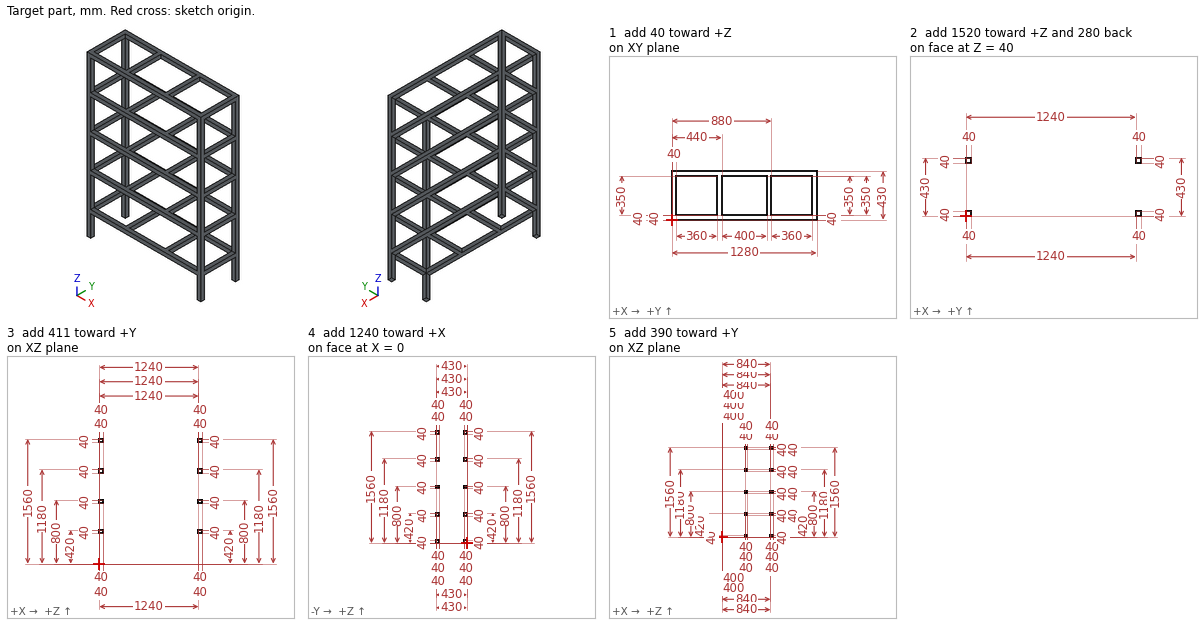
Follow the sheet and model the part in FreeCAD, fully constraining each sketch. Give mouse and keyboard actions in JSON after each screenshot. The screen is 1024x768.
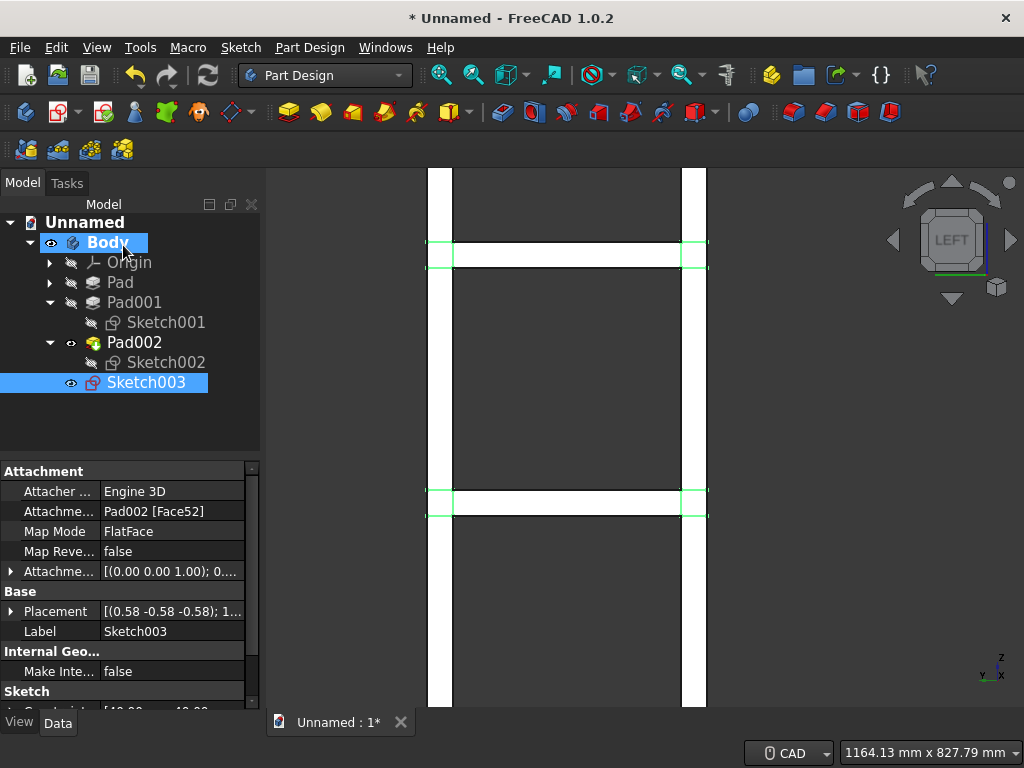
{"action": "left_click", "coordinate": [290, 112]}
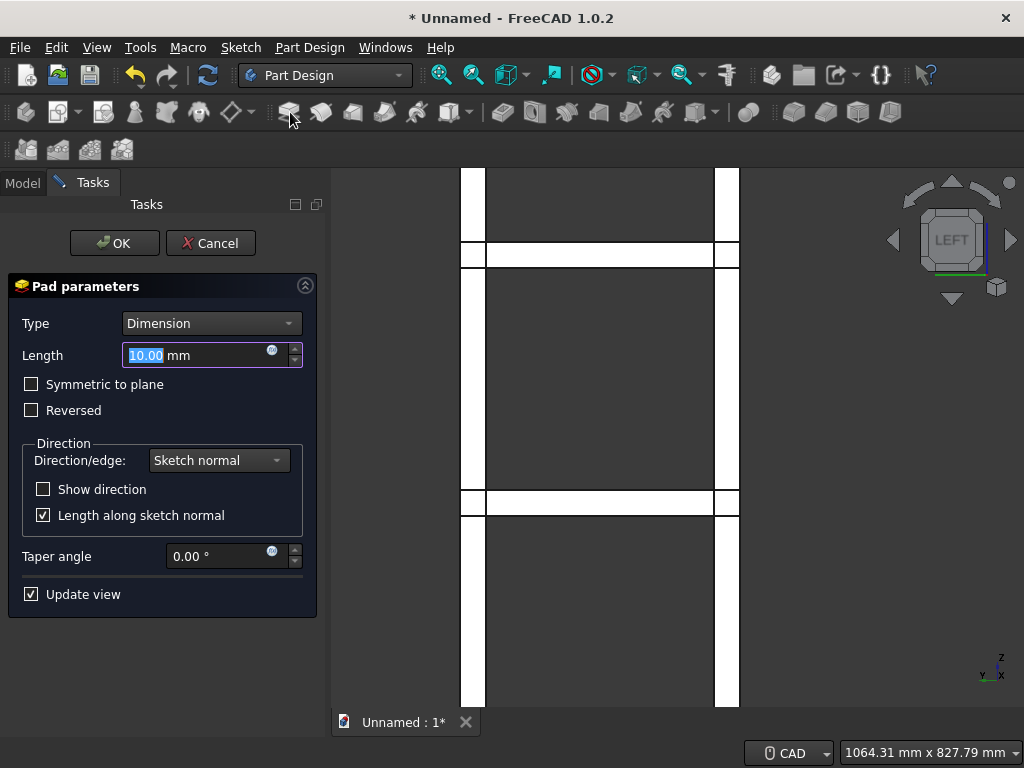
{"action": "type", "text": "1240"}
{"action": "key", "text": "Tab"}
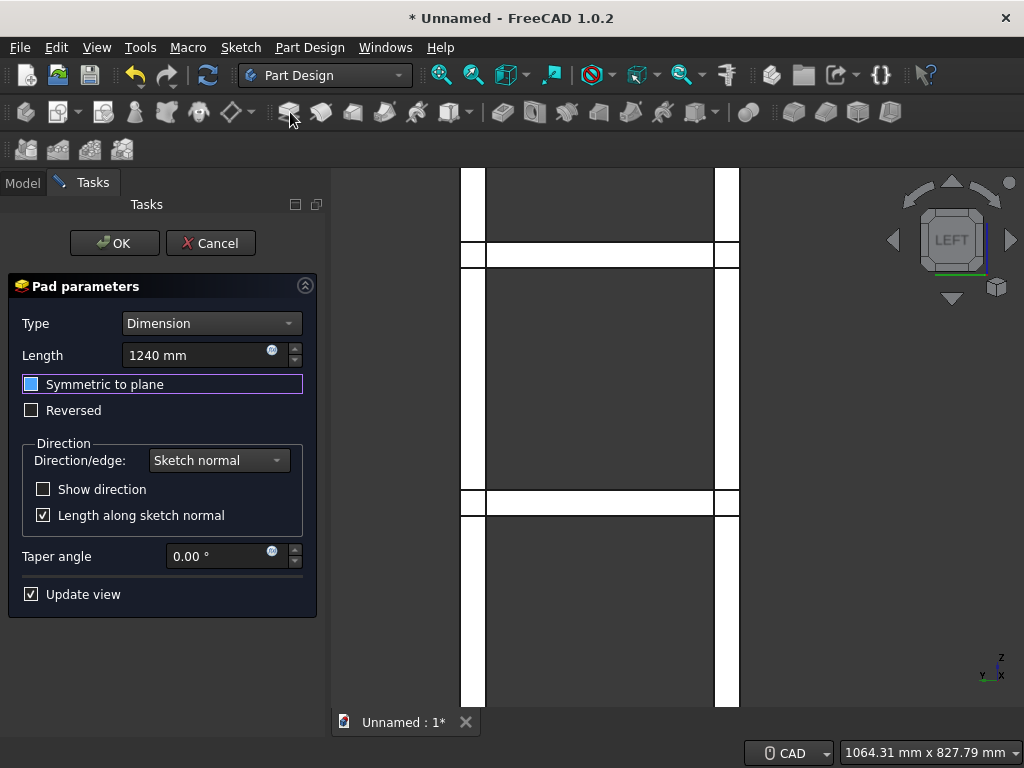
{"action": "left_click", "coordinate": [30, 410]}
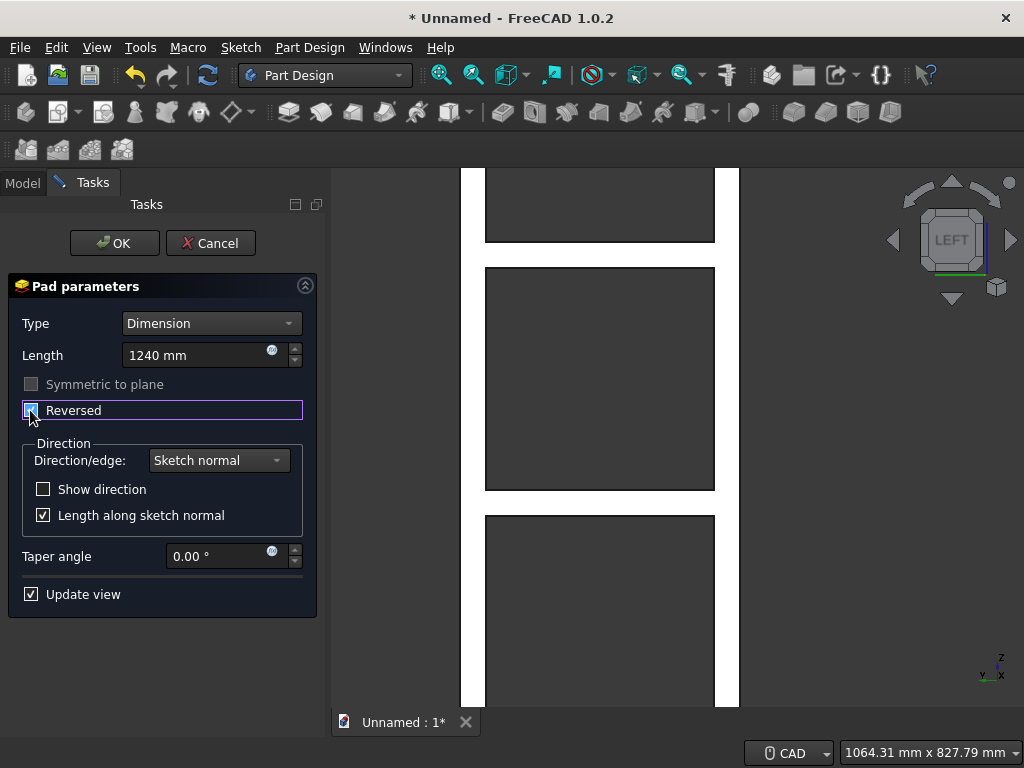
{"action": "left_click", "coordinate": [115, 243]}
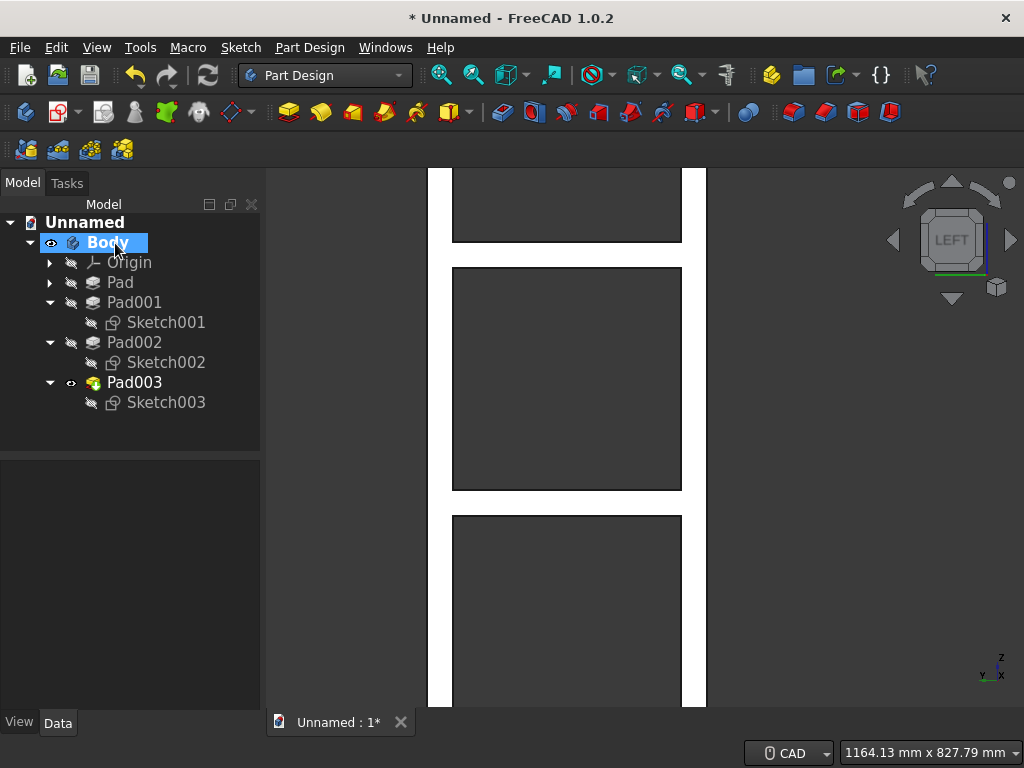
{"action": "left_click", "coordinate": [442, 76]}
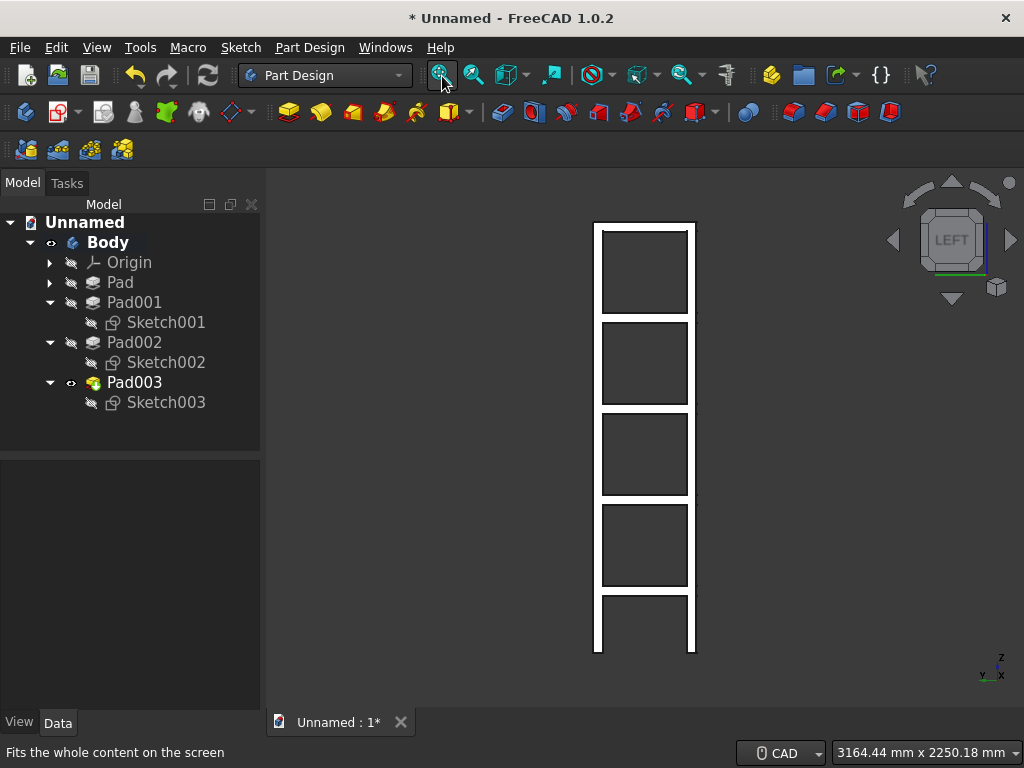
{"action": "left_click", "coordinate": [58, 112]}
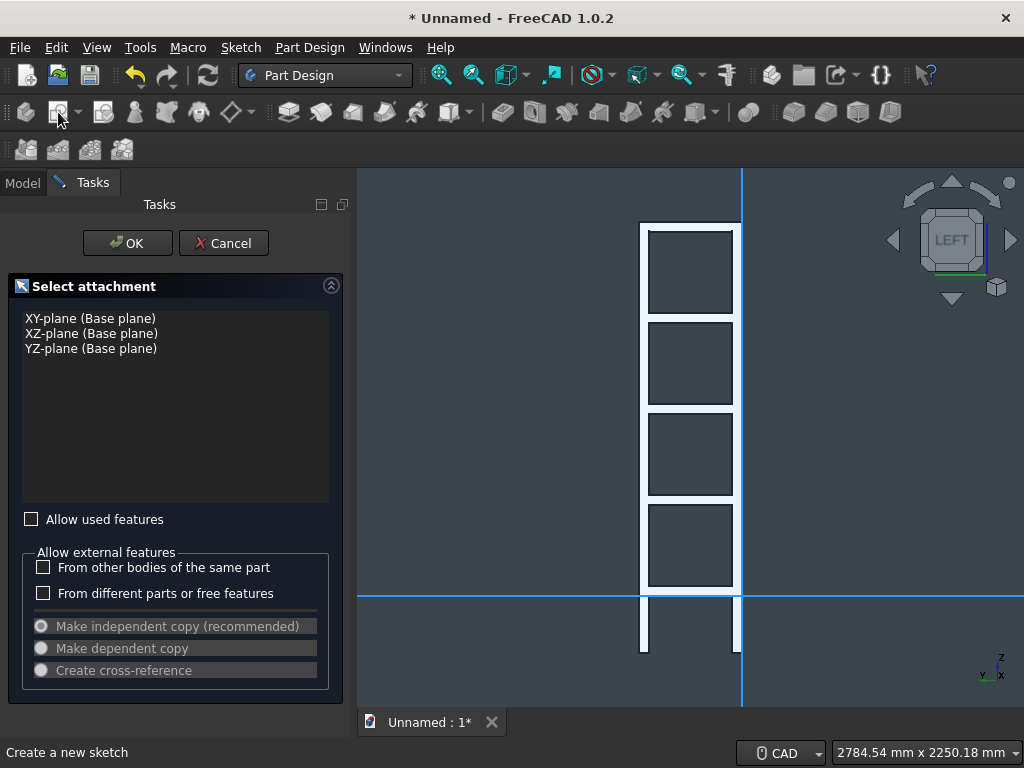
{"action": "left_click", "coordinate": [82, 334]}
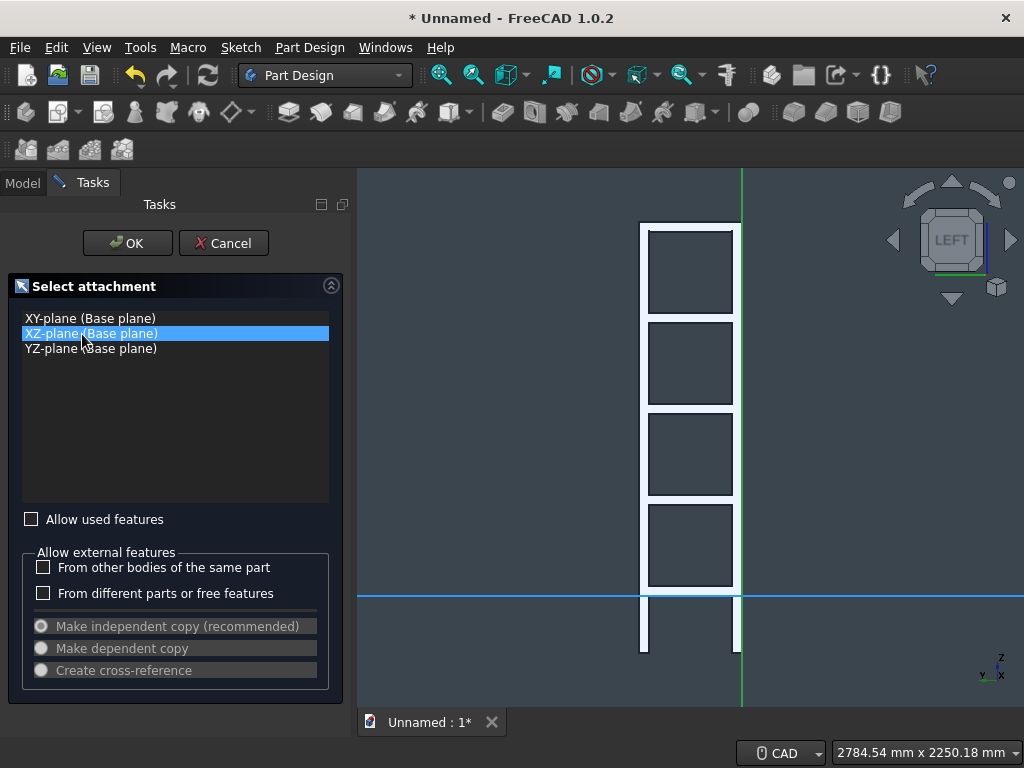
{"action": "left_click", "coordinate": [128, 243]}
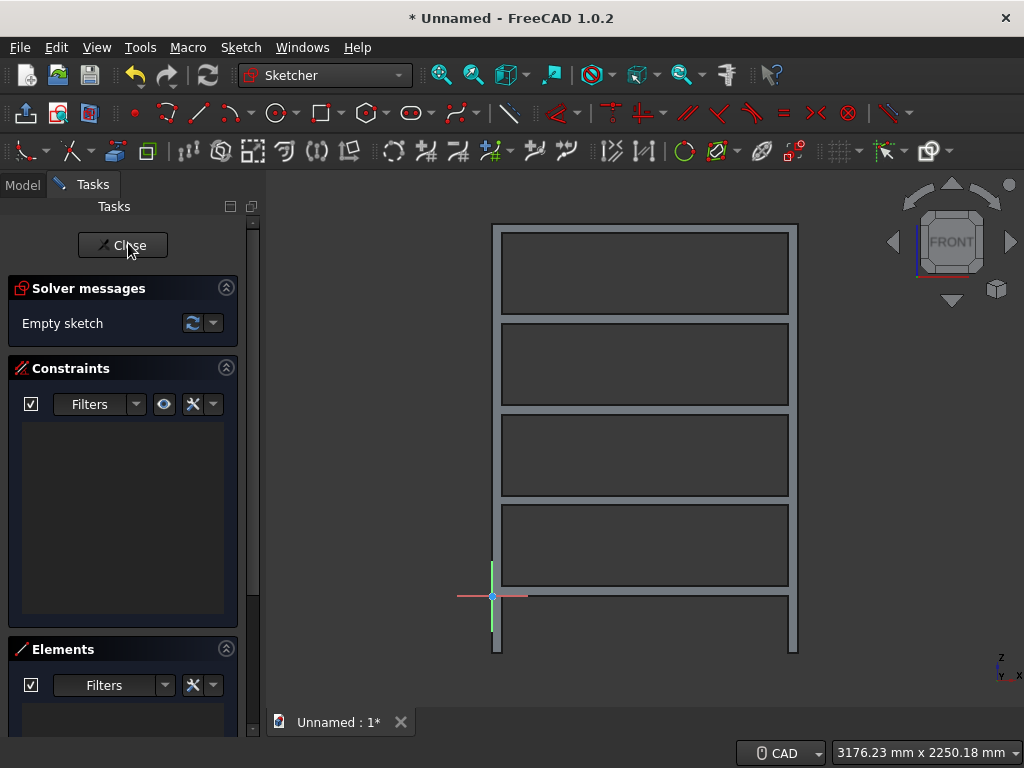
{"action": "left_click", "coordinate": [322, 114]}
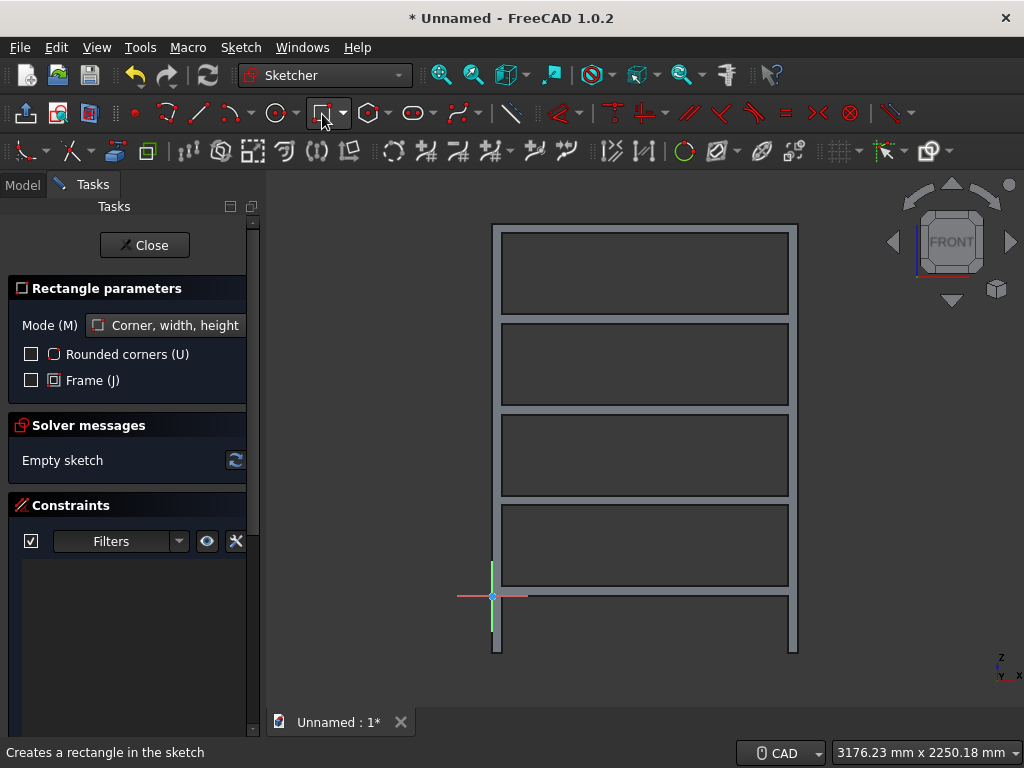
{"action": "scroll", "coordinate": [588, 586], "scroll_direction": "up", "scroll_amount": 3}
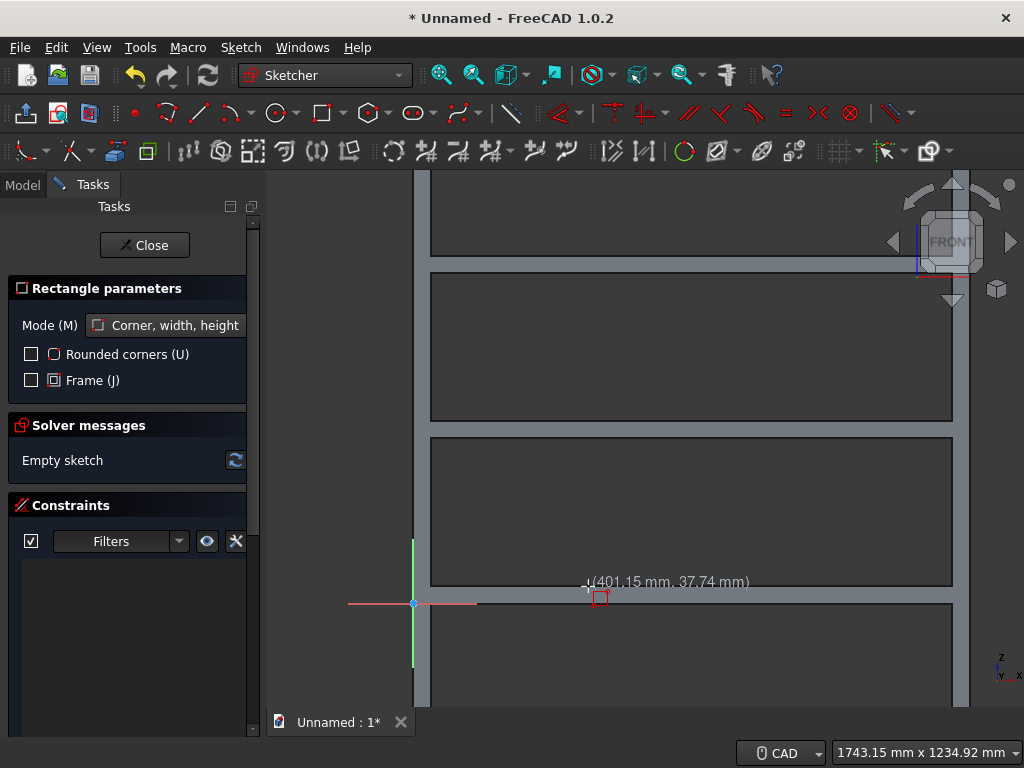
{"action": "left_click", "coordinate": [587, 586]}
{"action": "left_click", "coordinate": [605, 604]}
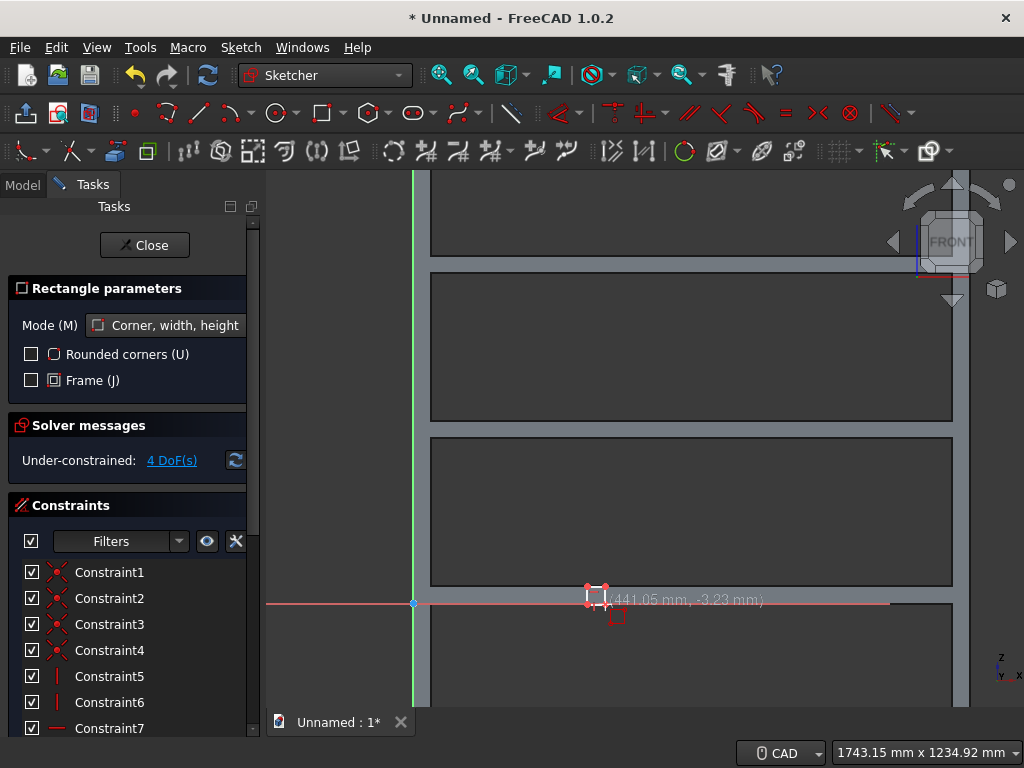
{"action": "left_click", "coordinate": [778, 586]}
{"action": "left_click", "coordinate": [796, 604]}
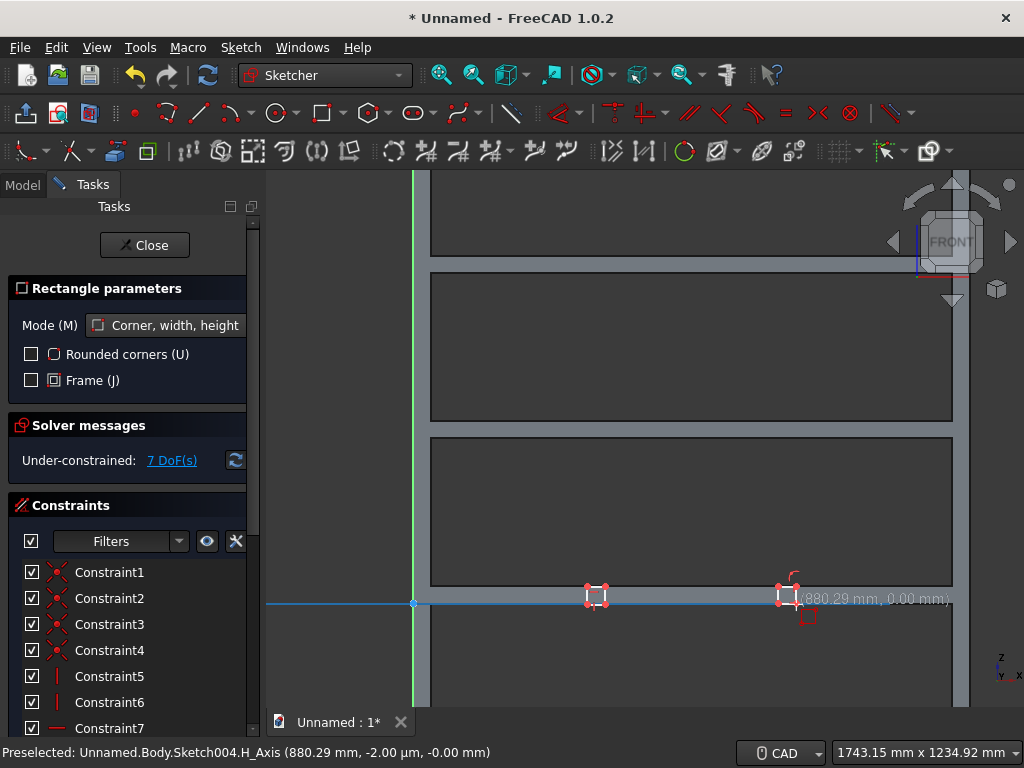
{"action": "left_click", "coordinate": [587, 421]}
{"action": "mouse_move", "coordinate": [605, 438]}